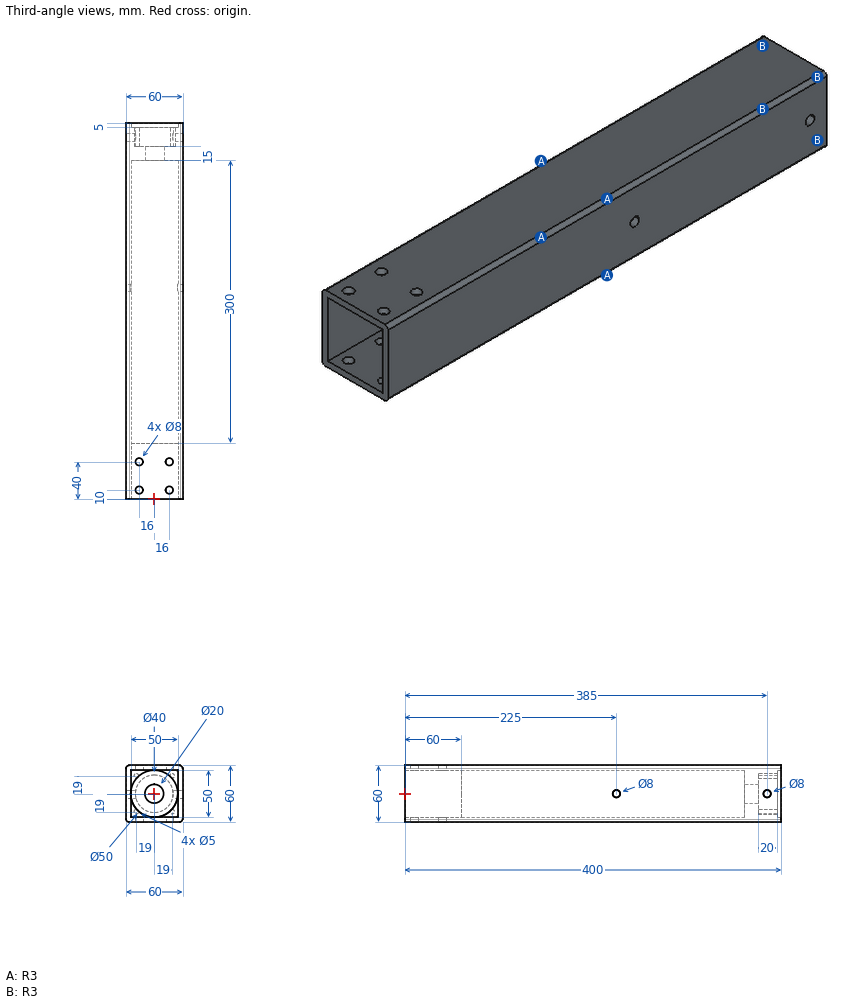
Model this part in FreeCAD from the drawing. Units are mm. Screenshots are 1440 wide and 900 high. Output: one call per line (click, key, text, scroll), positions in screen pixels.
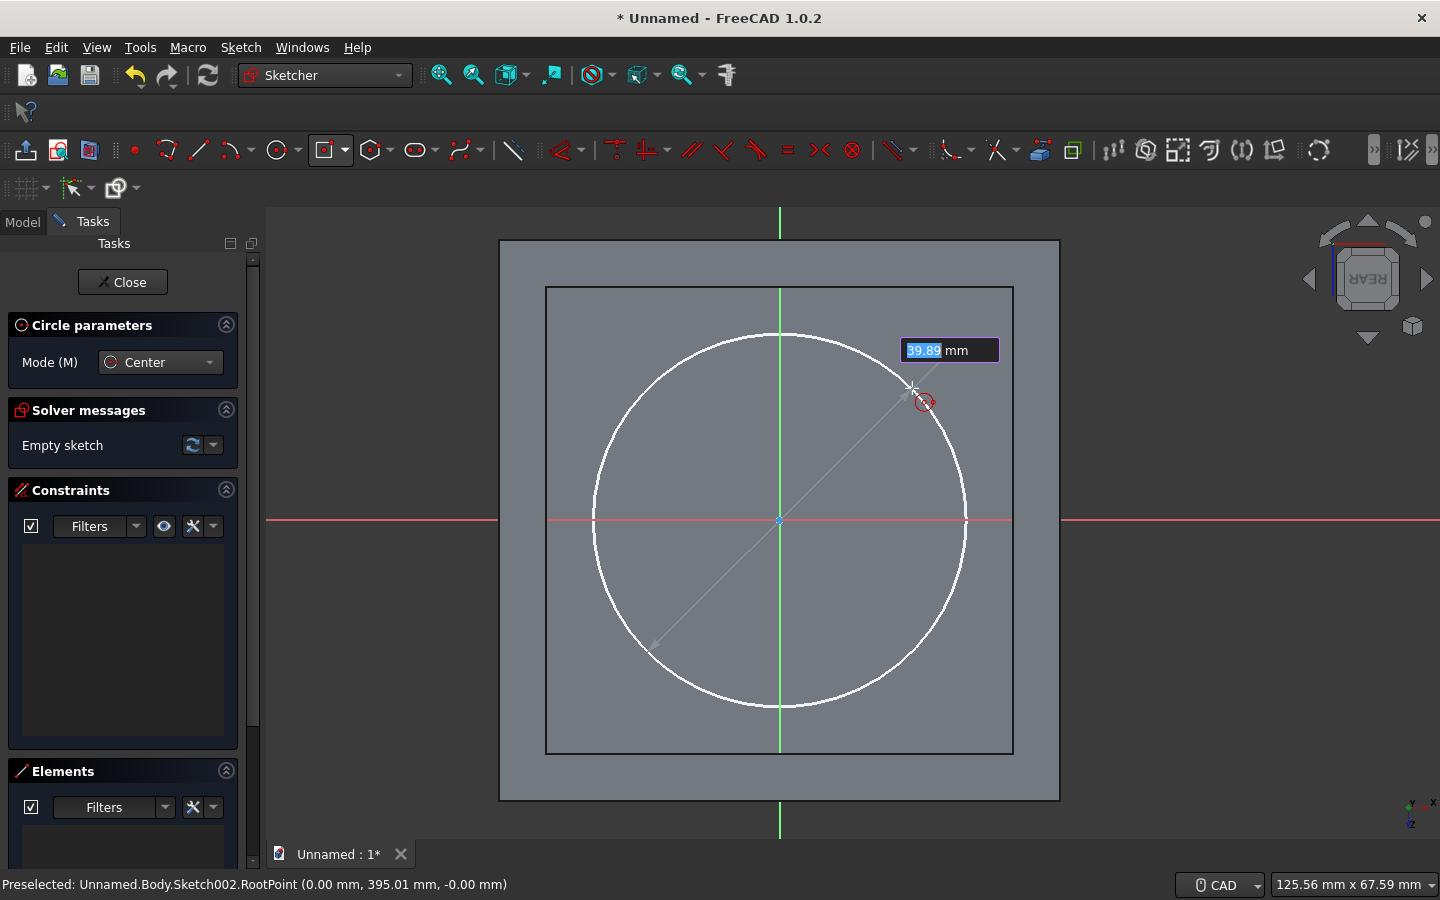
text(40)
key(Return)
key(Escape)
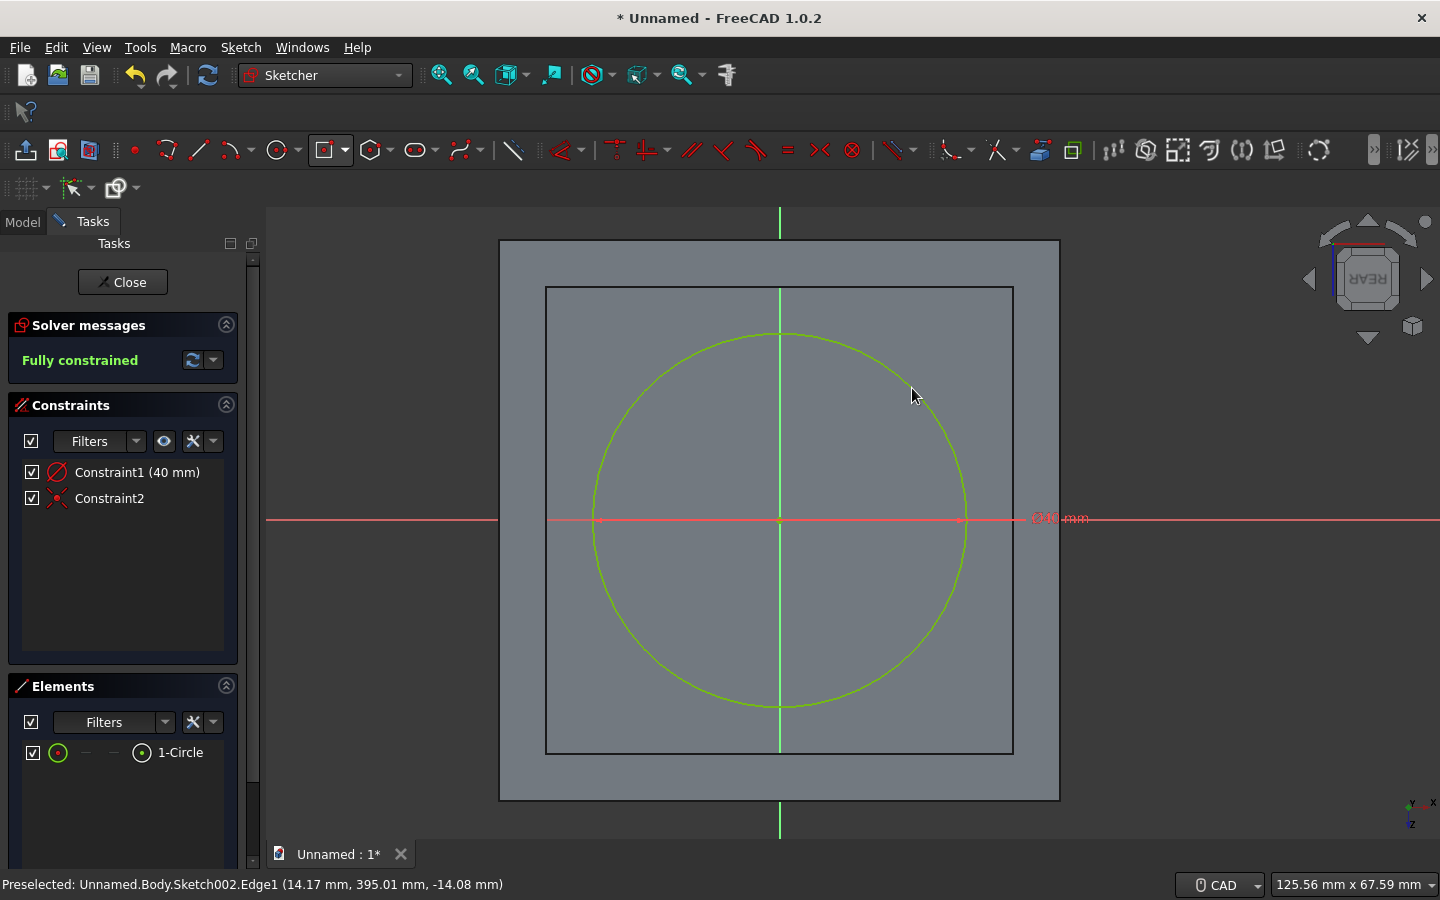
click(123, 282)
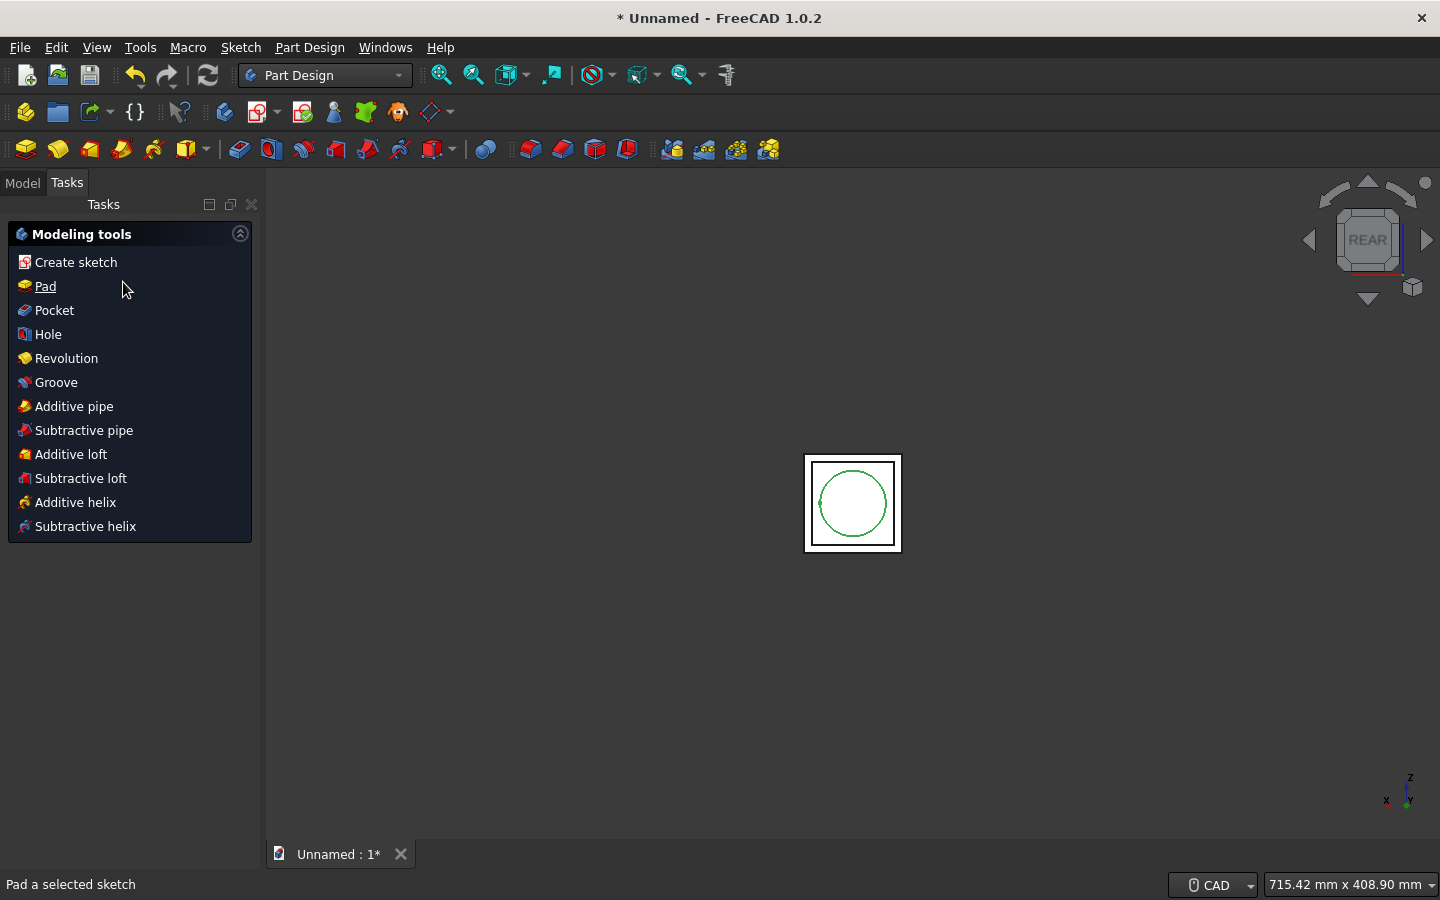
click(240, 150)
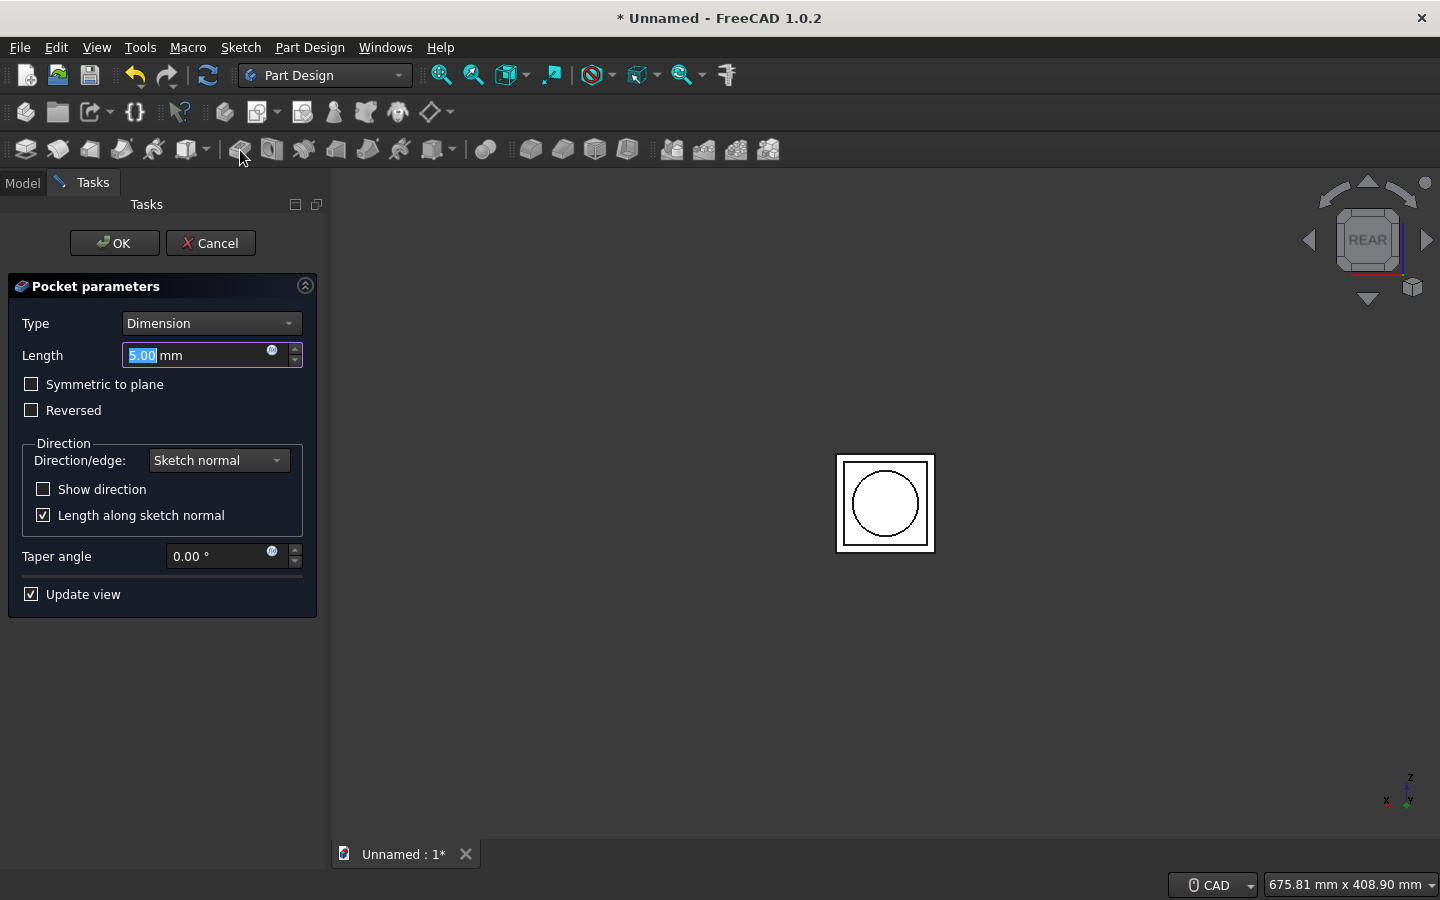
text(20)
key(Tab)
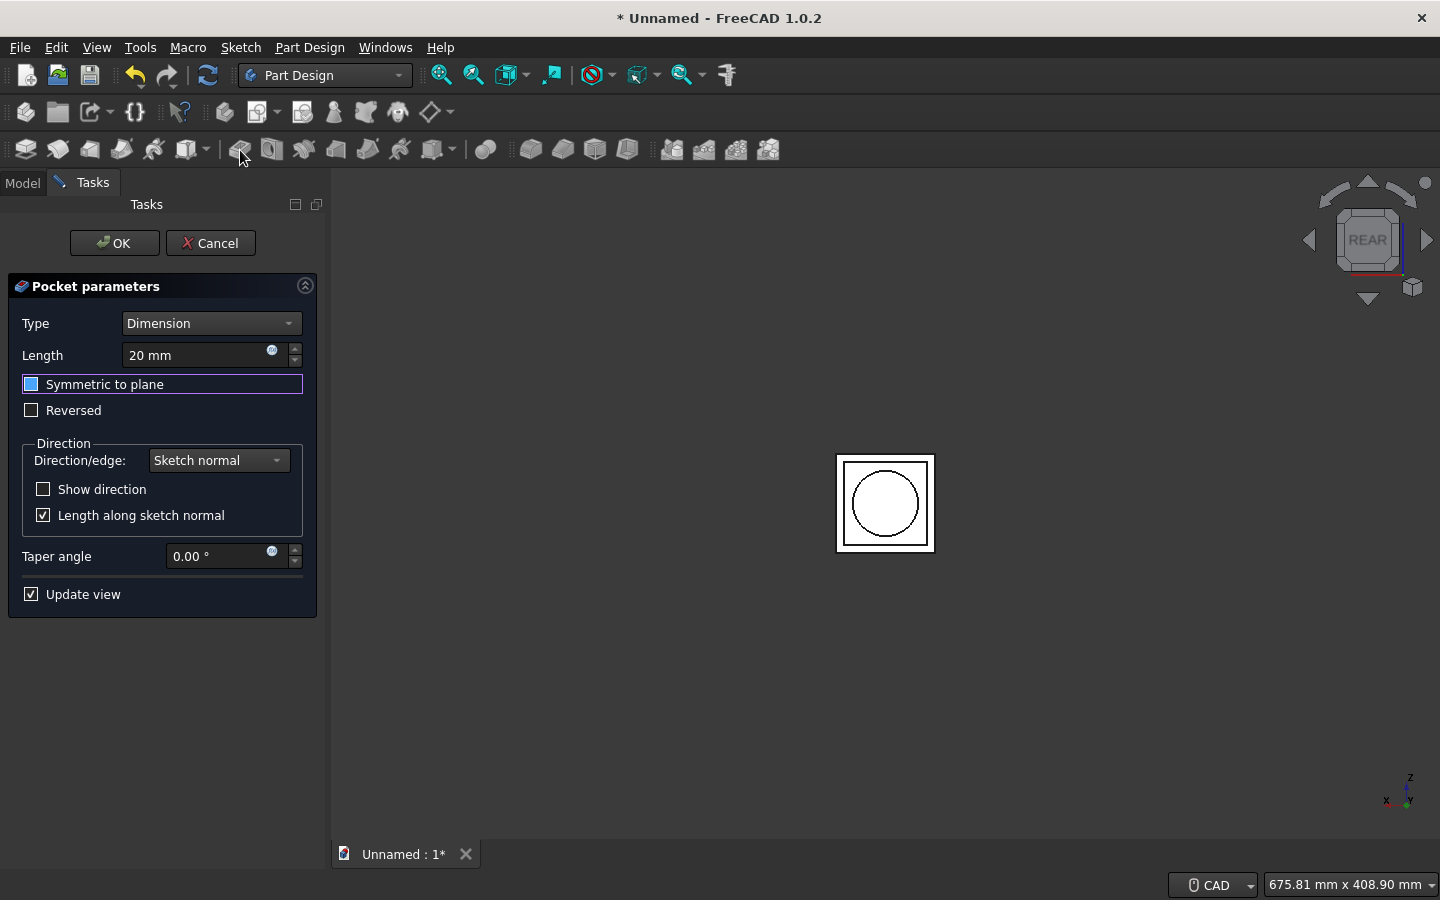
click(115, 243)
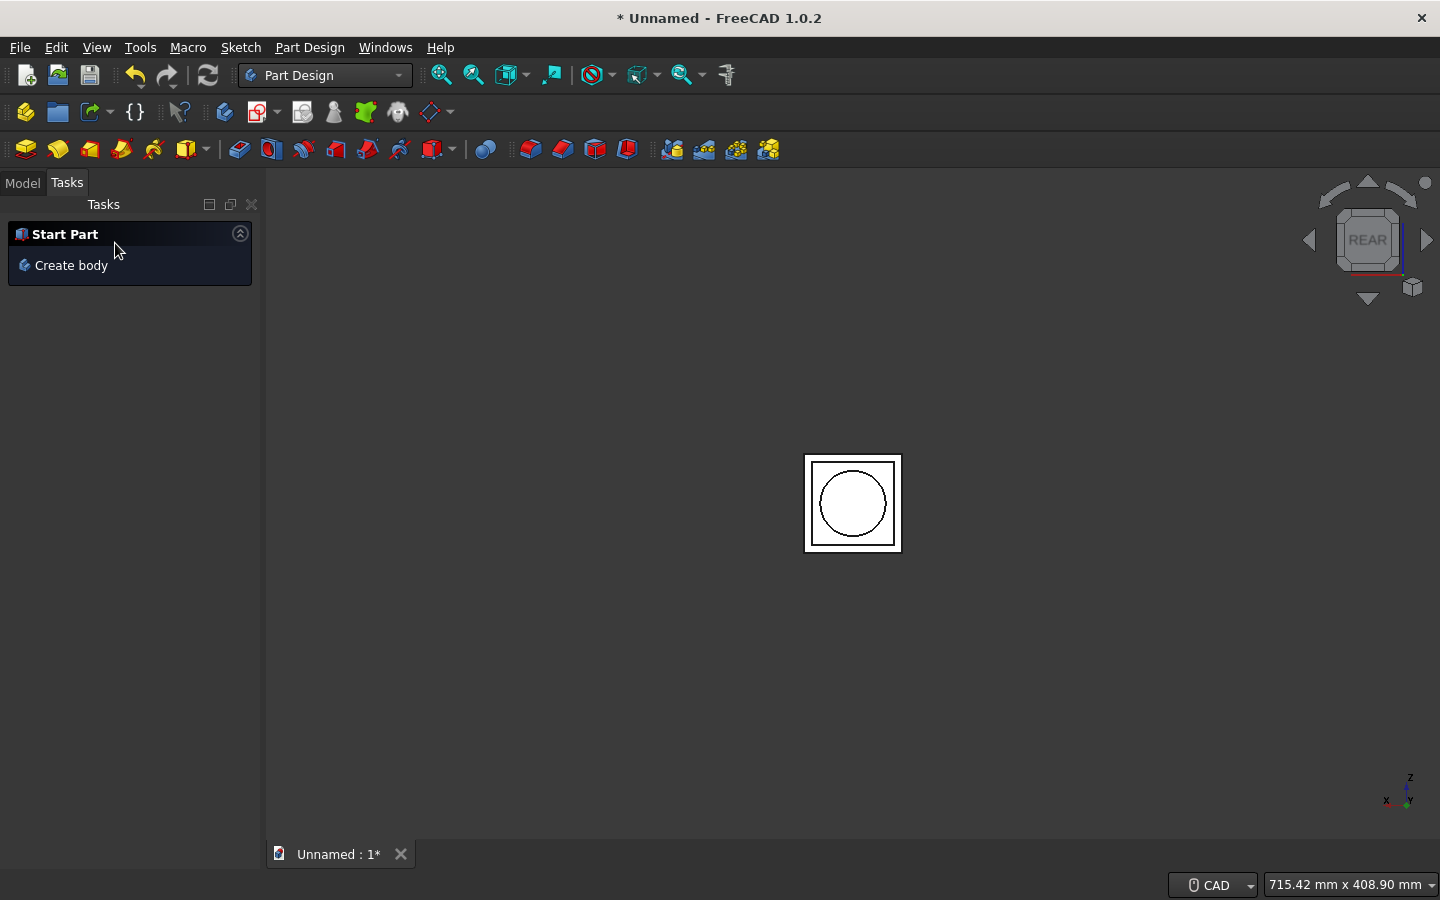
click(442, 76)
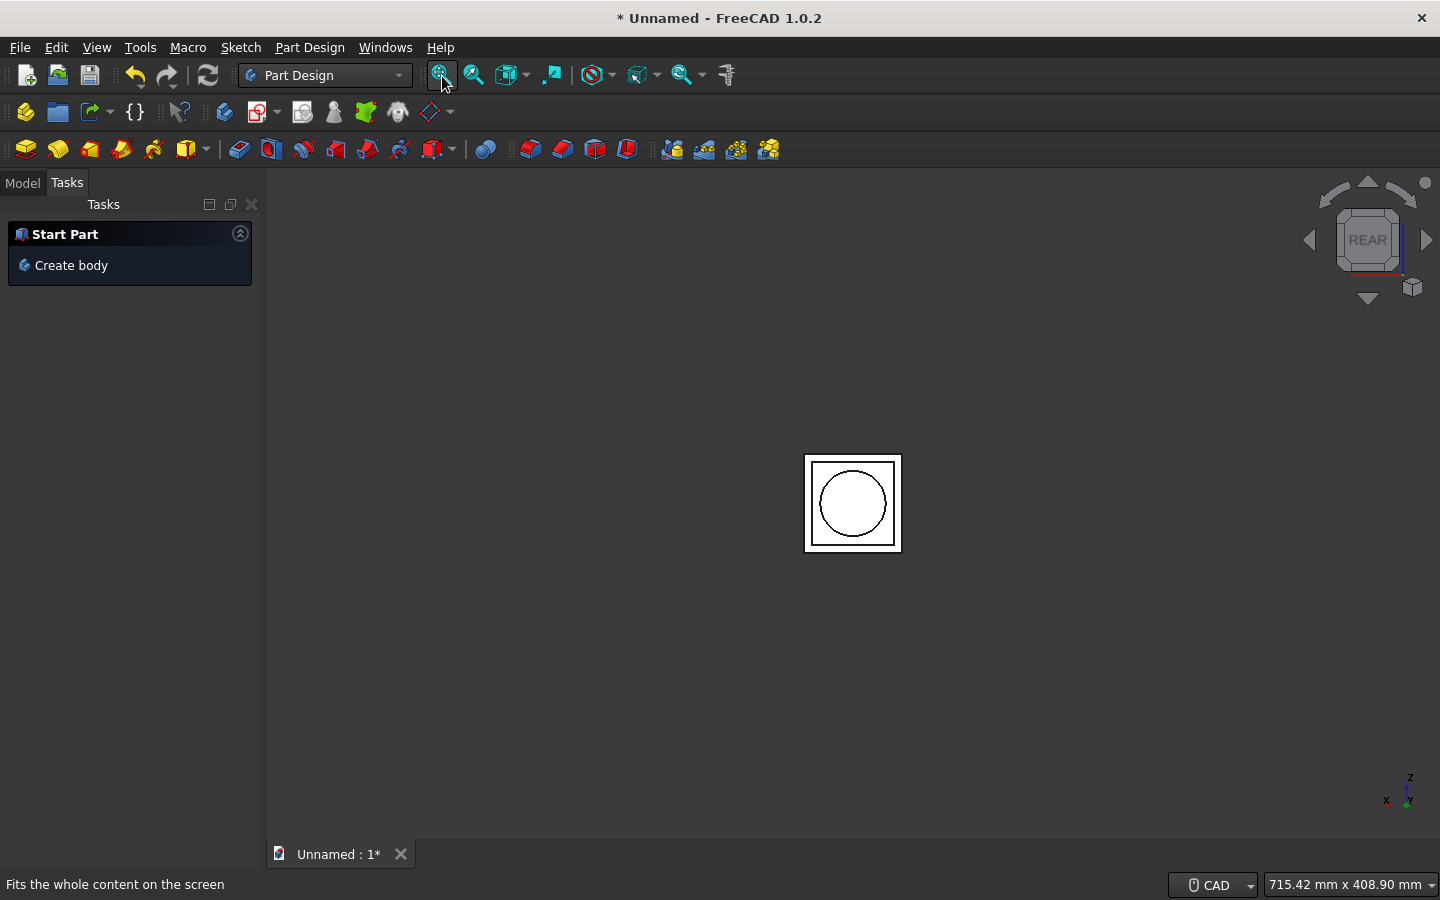
click(853, 502)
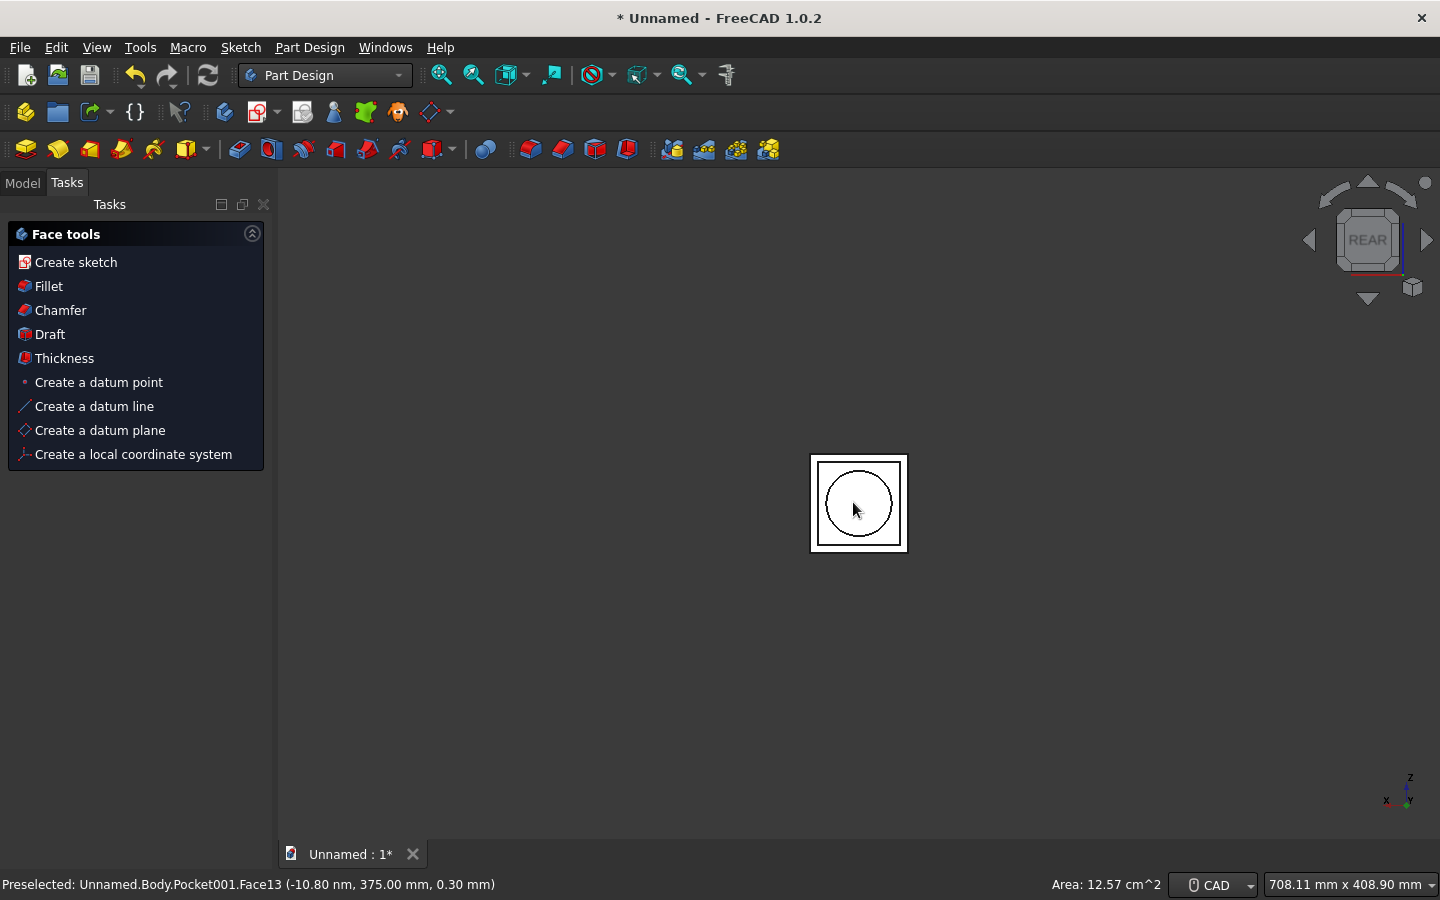
click(258, 112)